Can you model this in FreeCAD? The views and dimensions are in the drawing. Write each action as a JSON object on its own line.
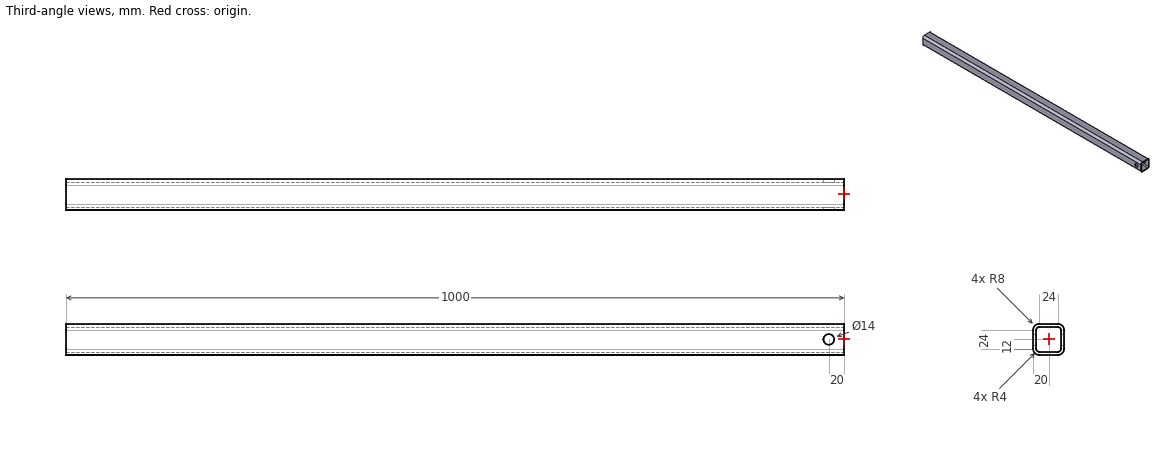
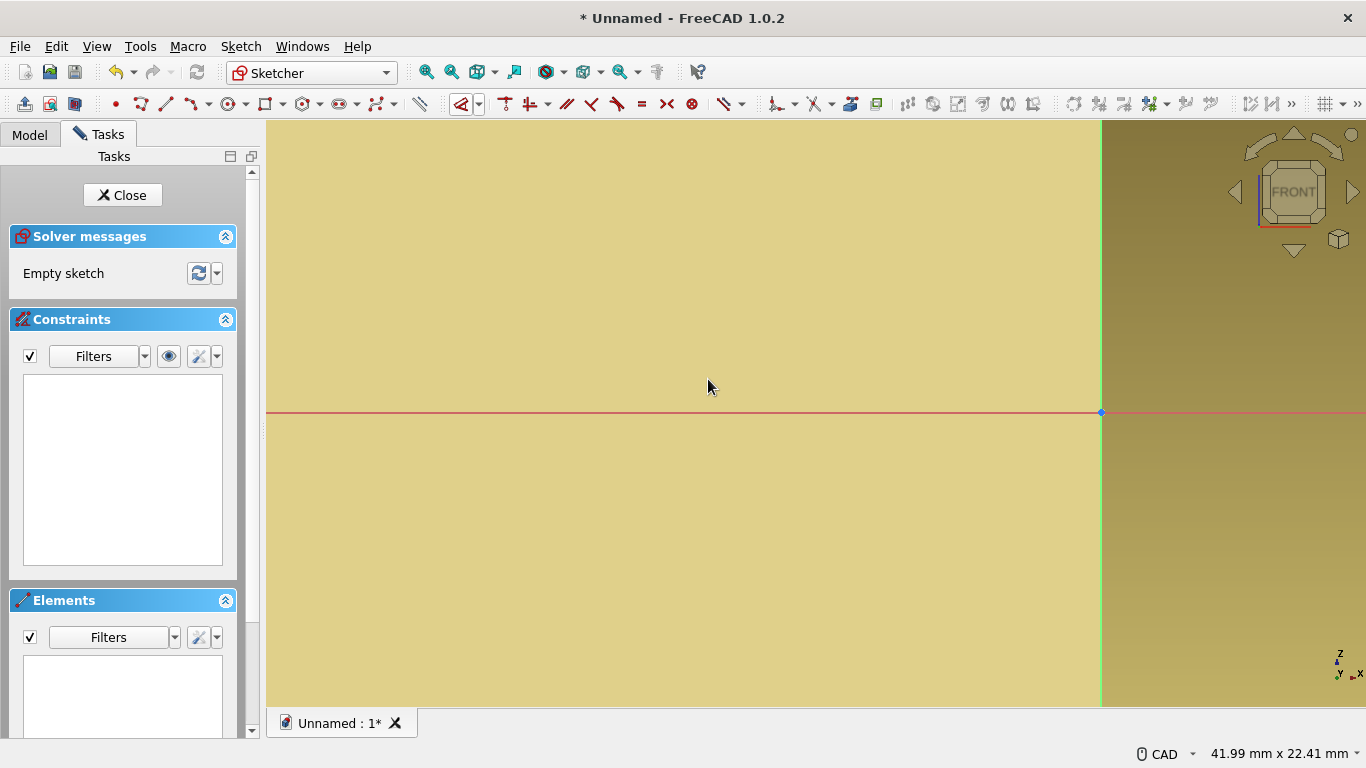
{"action": "left_click", "coordinate": [228, 104]}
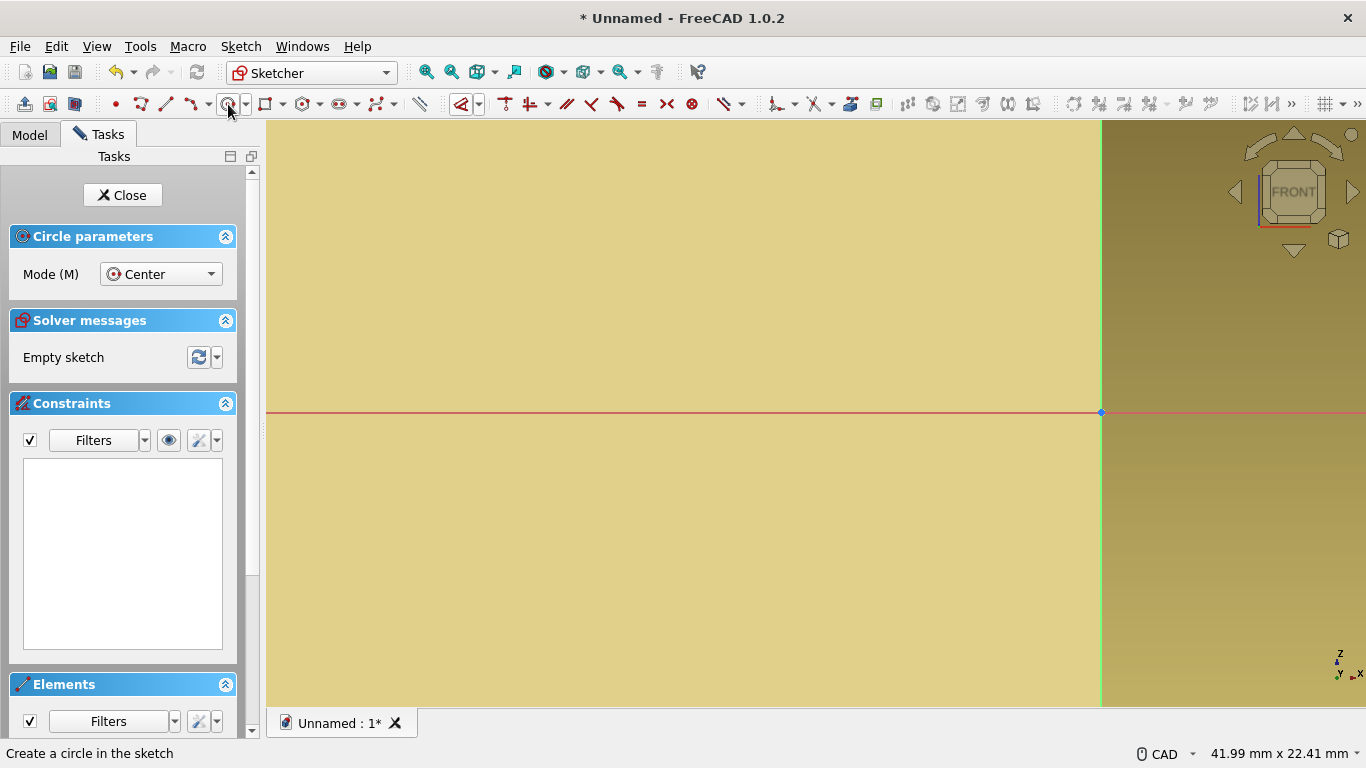
{"action": "left_click", "coordinate": [577, 413]}
{"action": "mouse_move", "coordinate": [707, 283]}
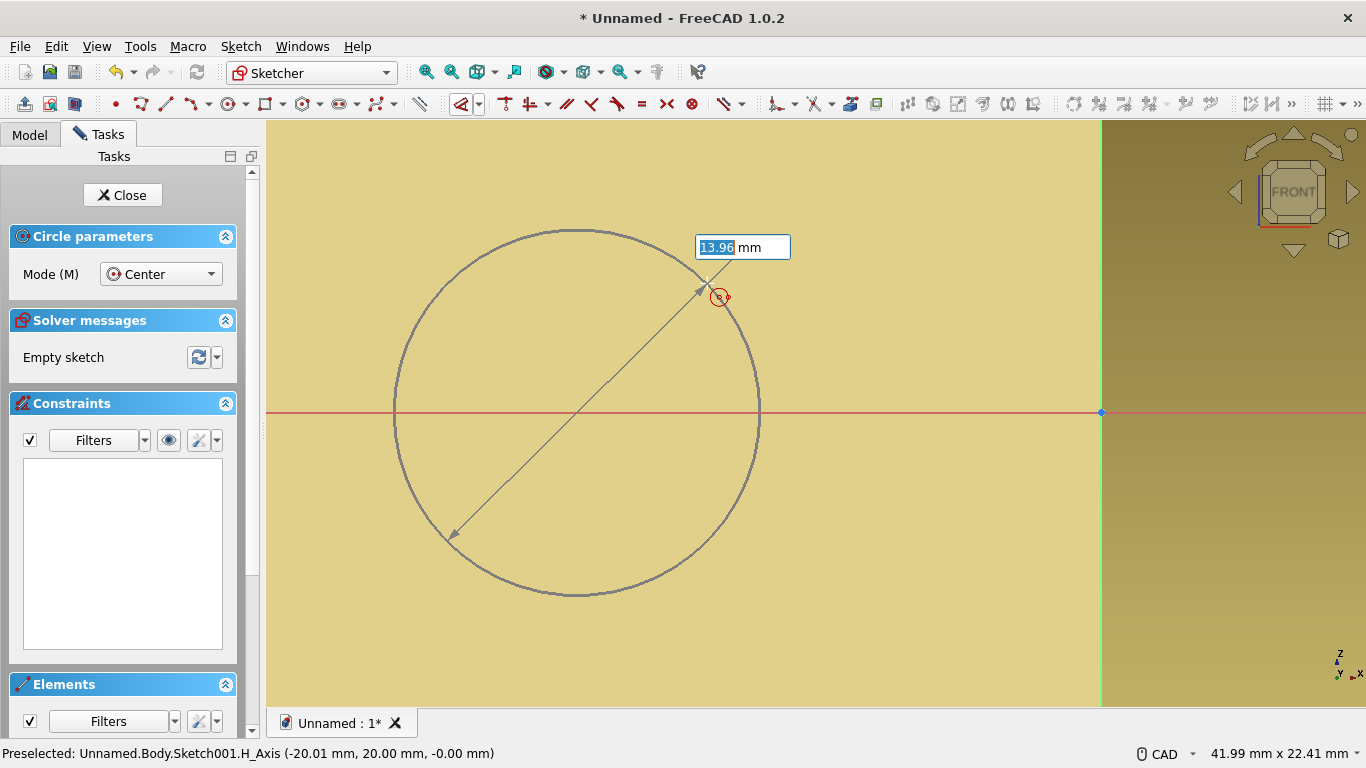
{"action": "type", "text": "14"}
{"action": "key", "text": "Return"}
{"action": "key", "text": "Escape"}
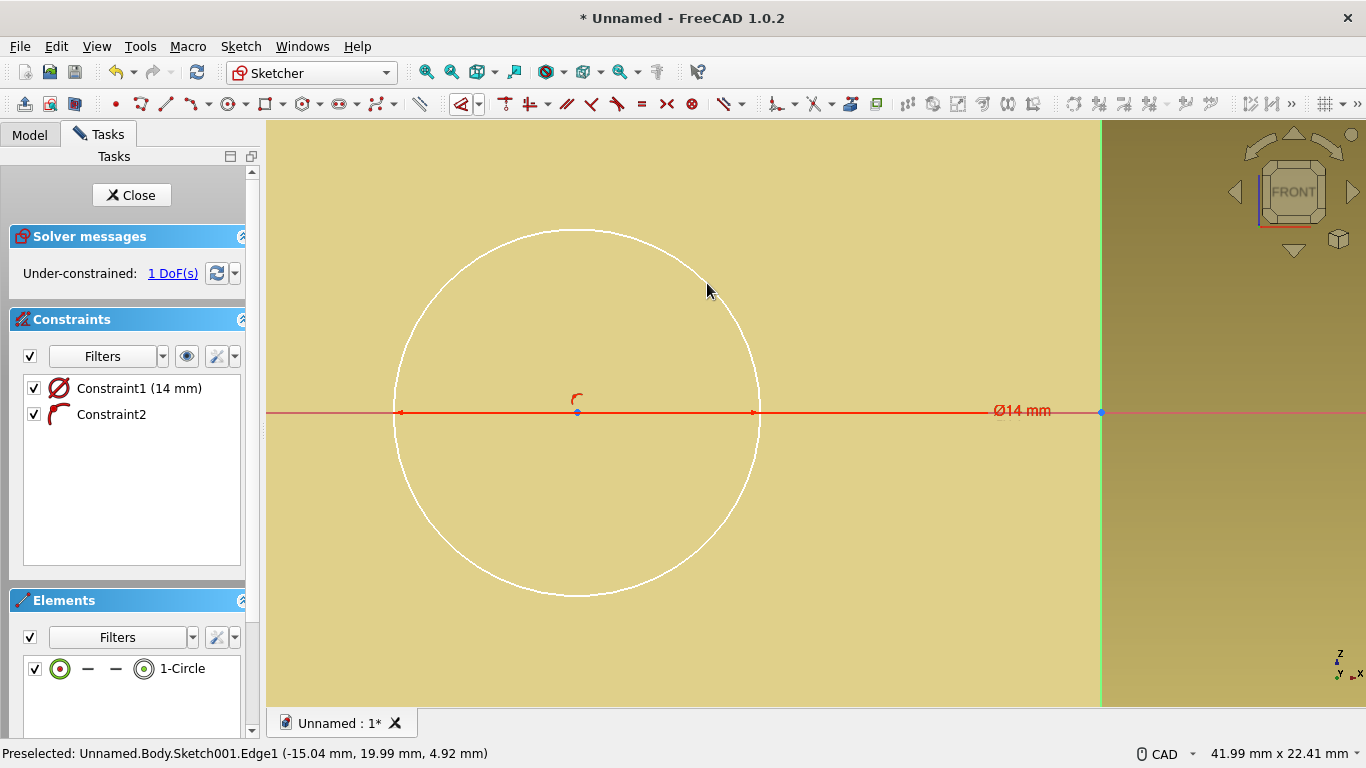
{"action": "left_click", "coordinate": [577, 413]}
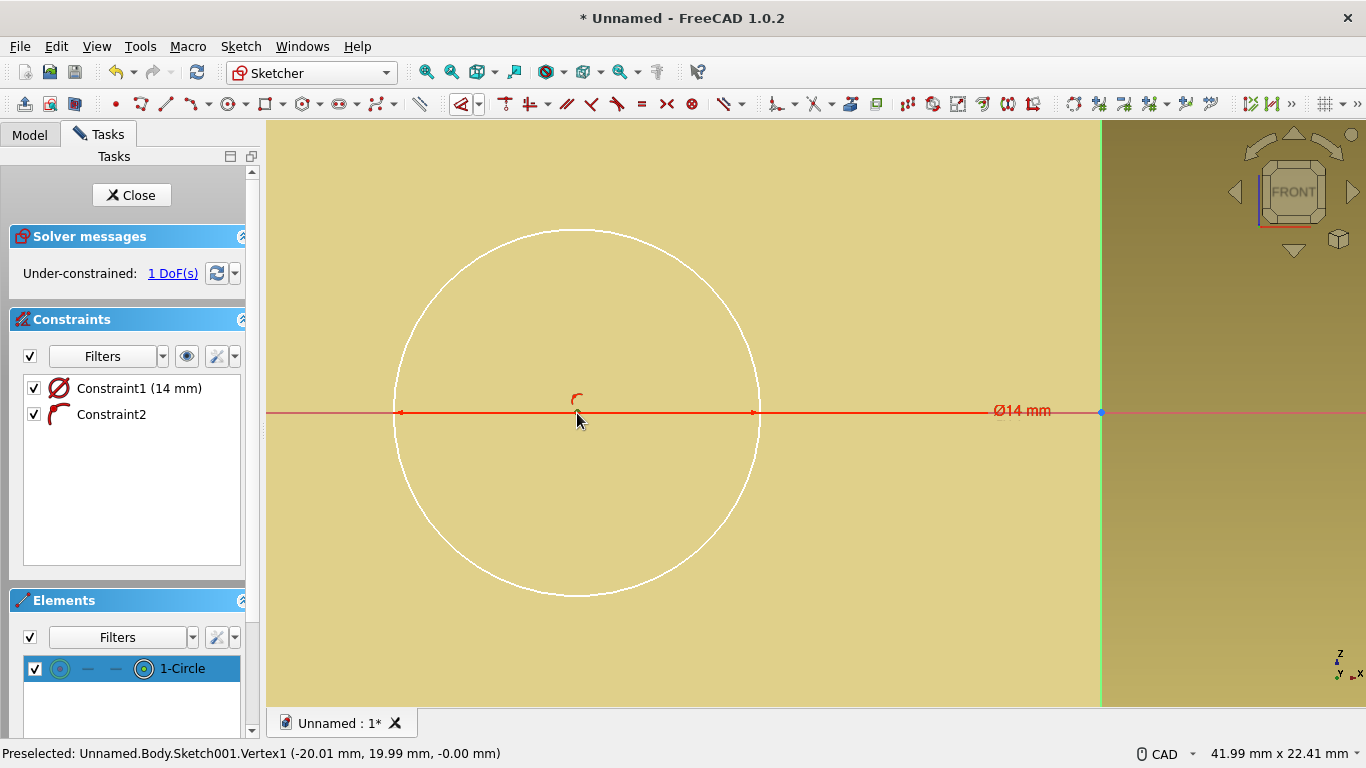
{"action": "key", "text": "l"}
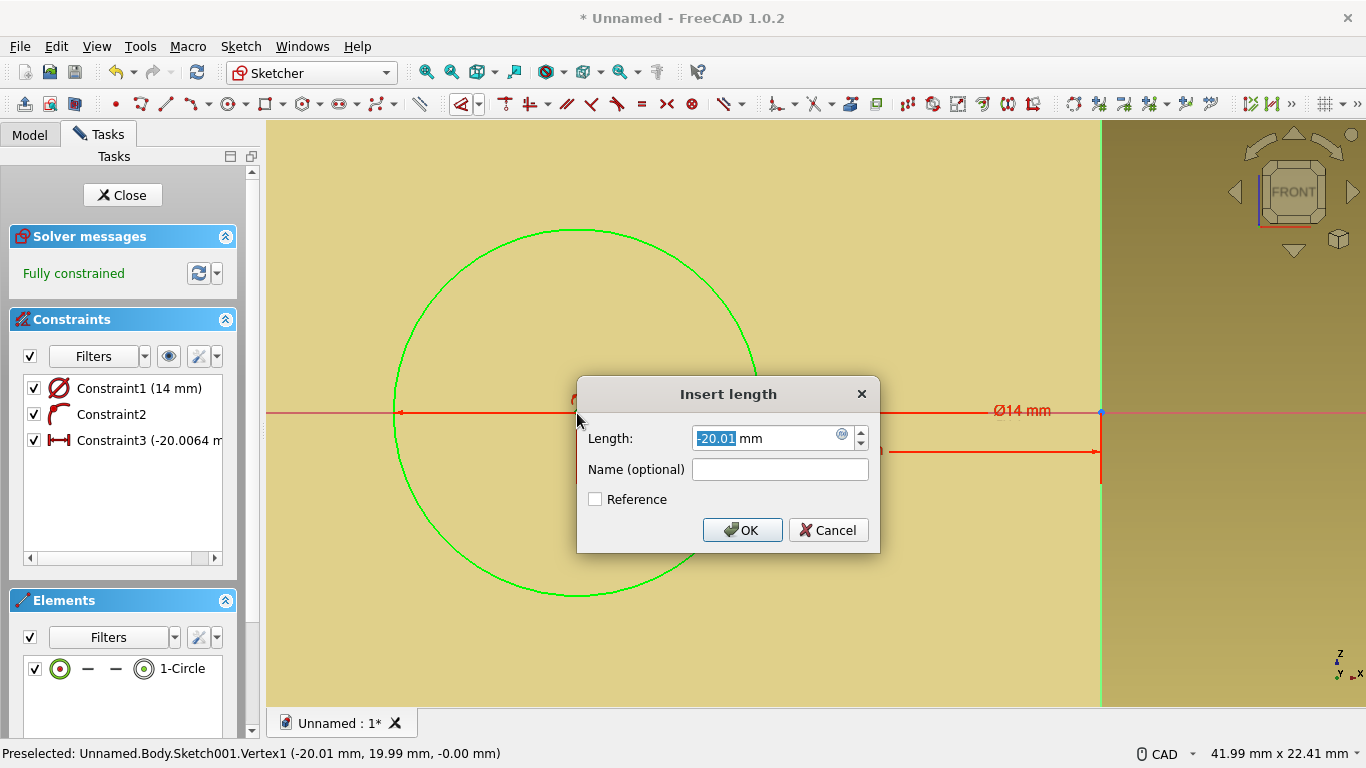
{"action": "type", "text": "-20"}
{"action": "key", "text": "Return"}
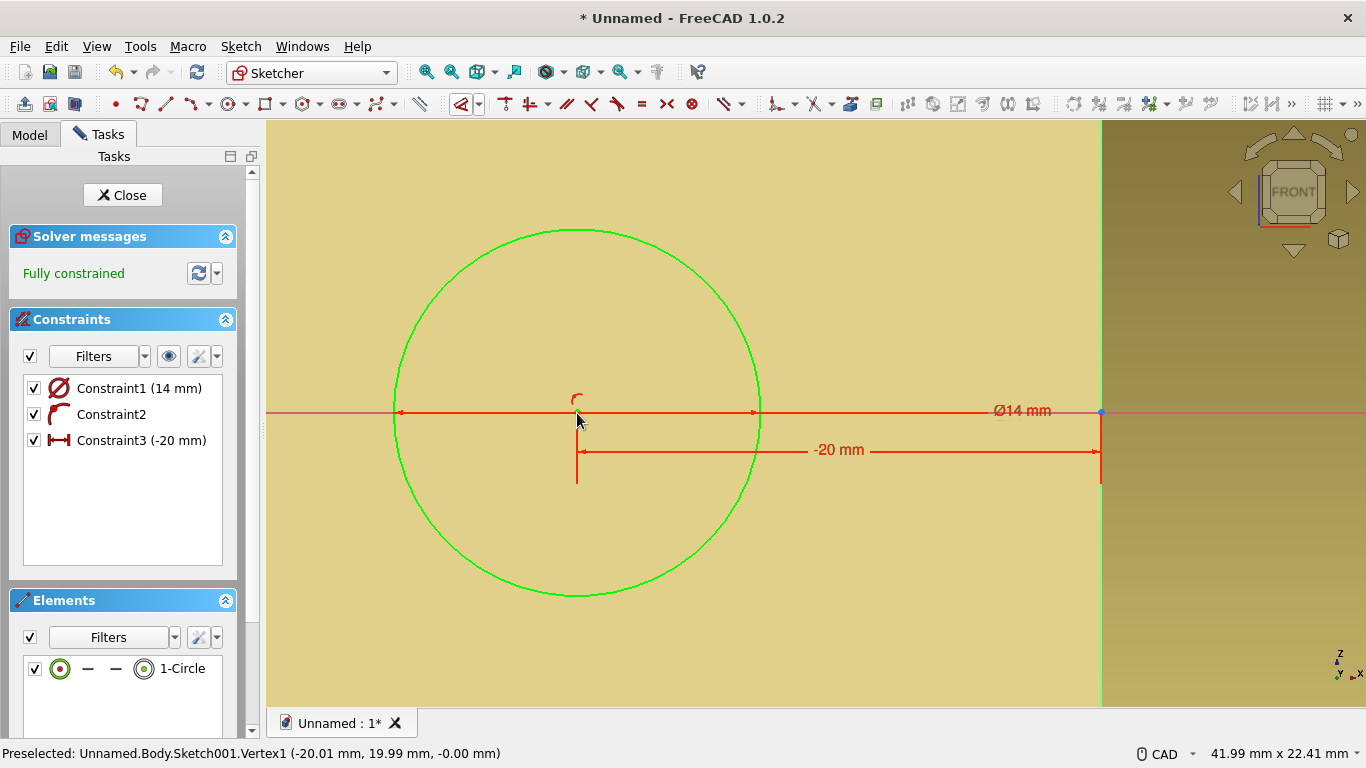
{"action": "left_click", "coordinate": [123, 195]}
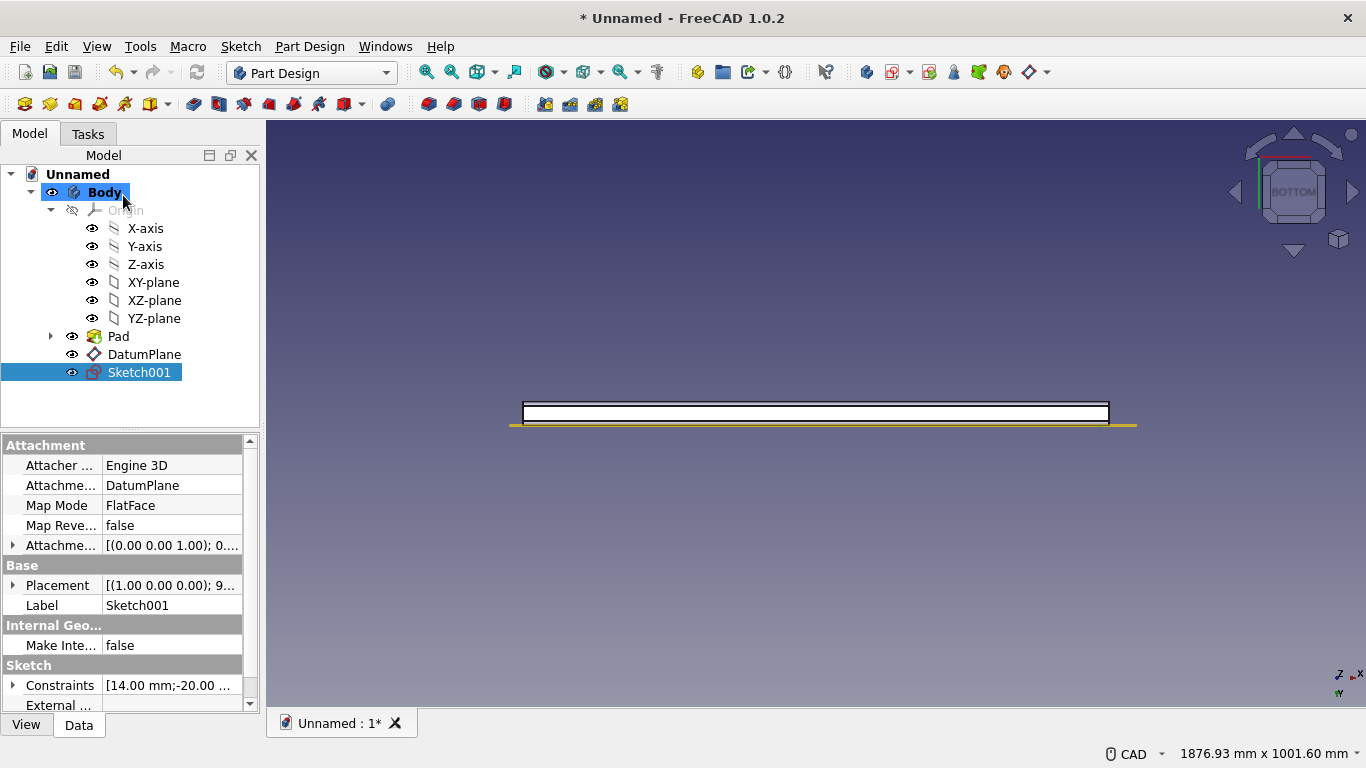
{"action": "left_click", "coordinate": [194, 104]}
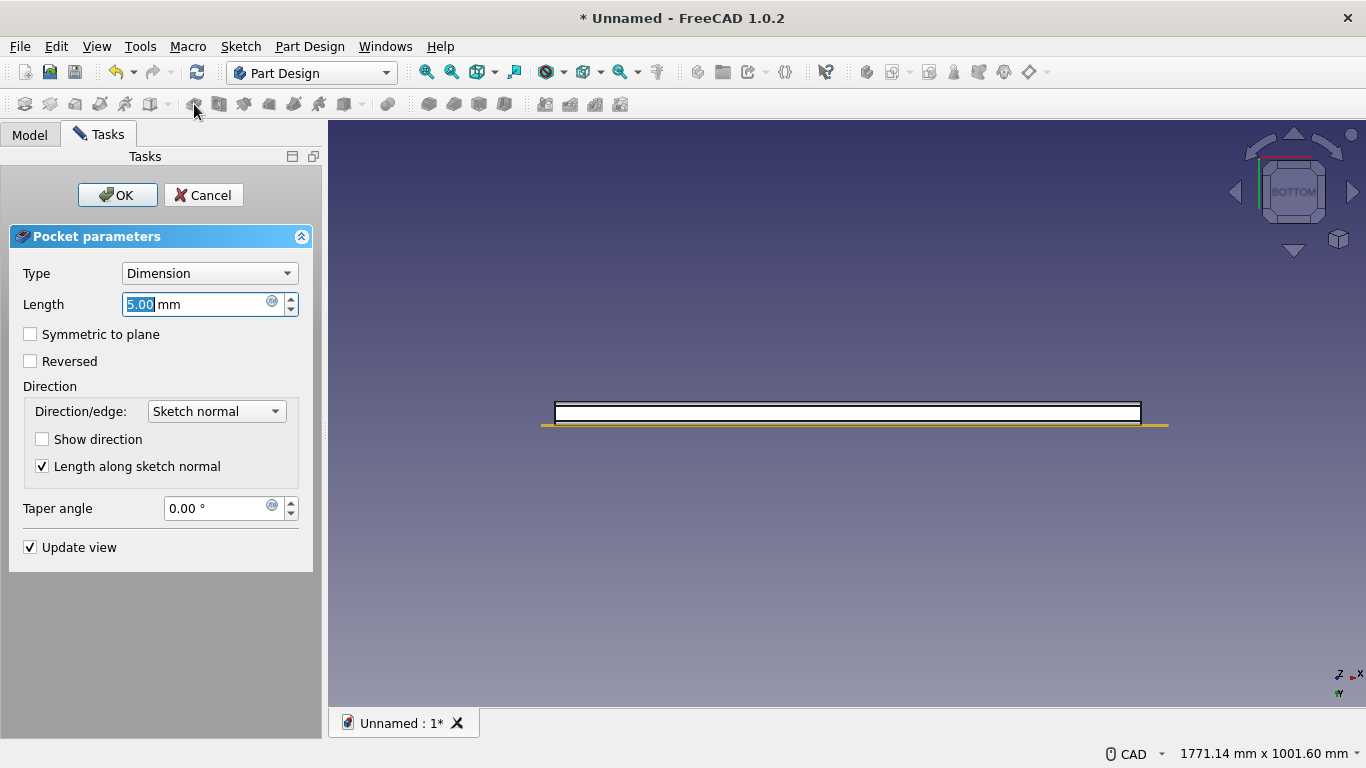
{"action": "left_click", "coordinate": [210, 274]}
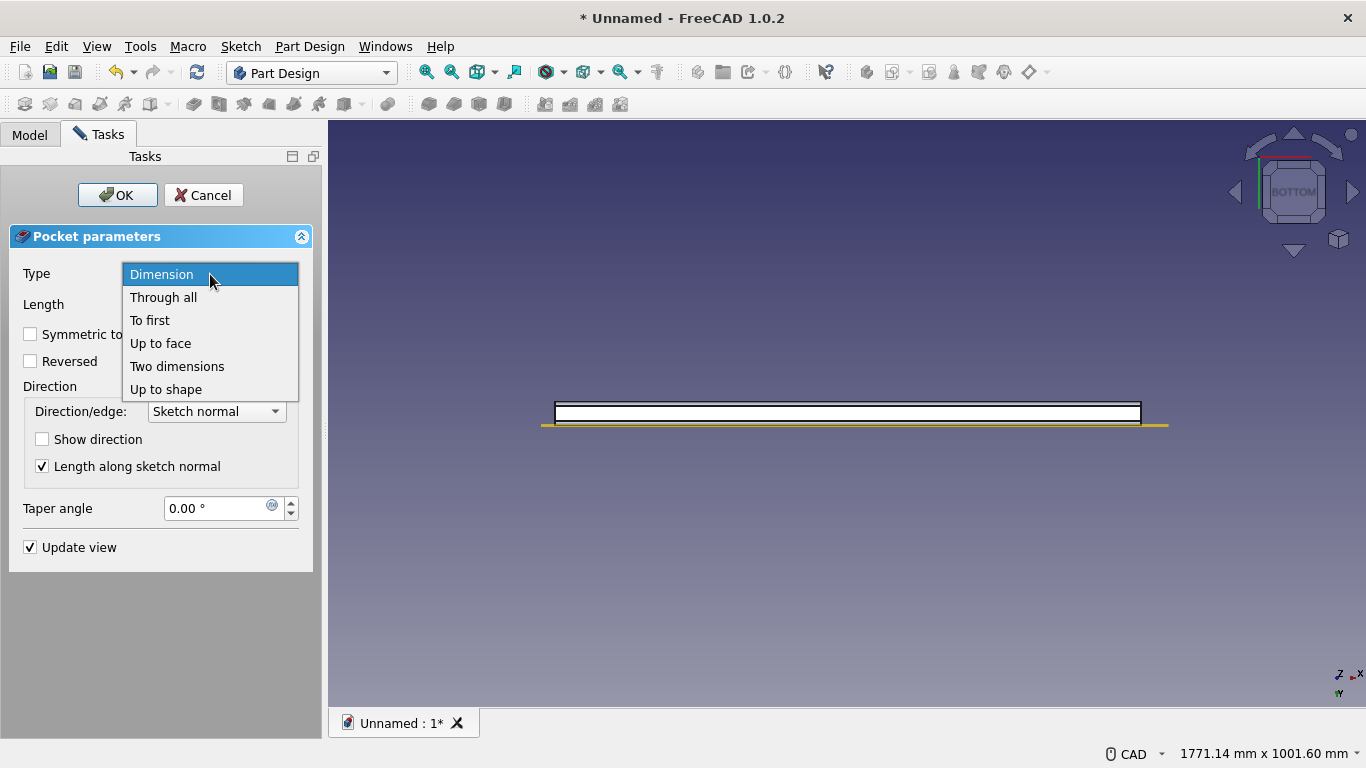
{"action": "left_click", "coordinate": [208, 298]}